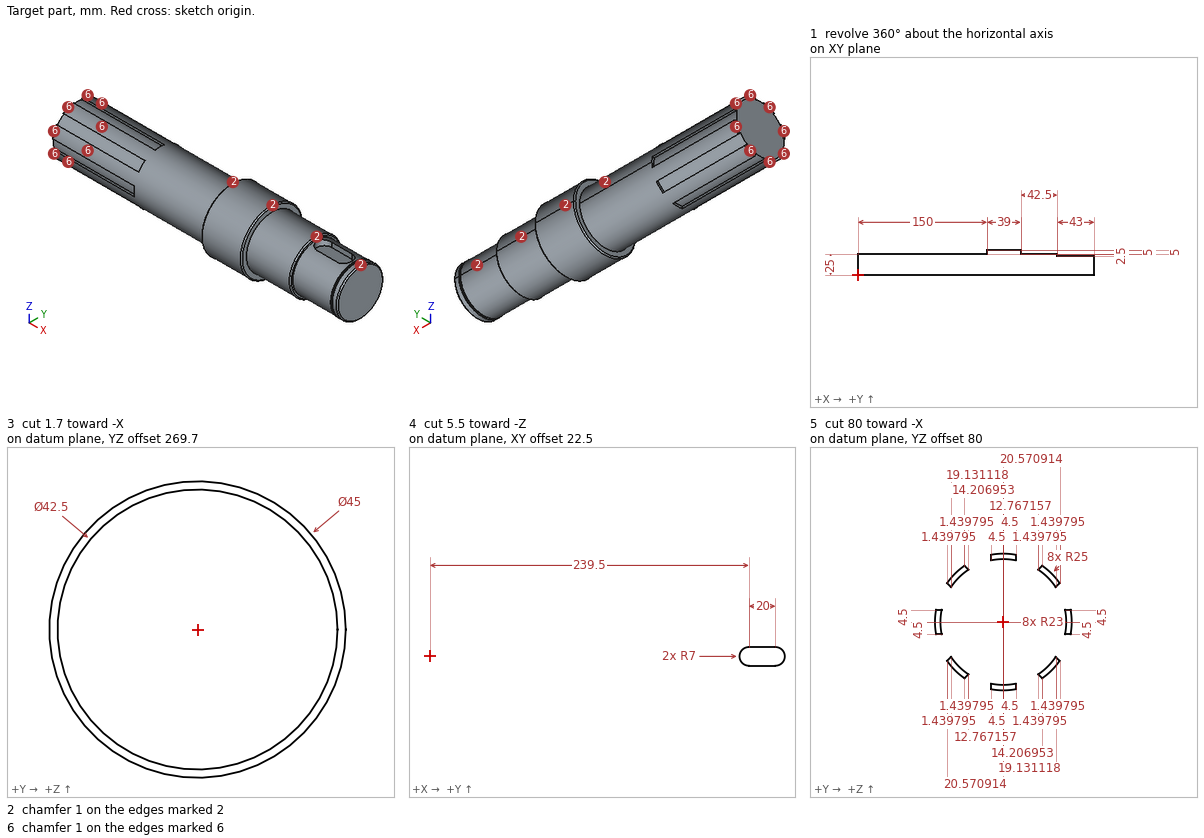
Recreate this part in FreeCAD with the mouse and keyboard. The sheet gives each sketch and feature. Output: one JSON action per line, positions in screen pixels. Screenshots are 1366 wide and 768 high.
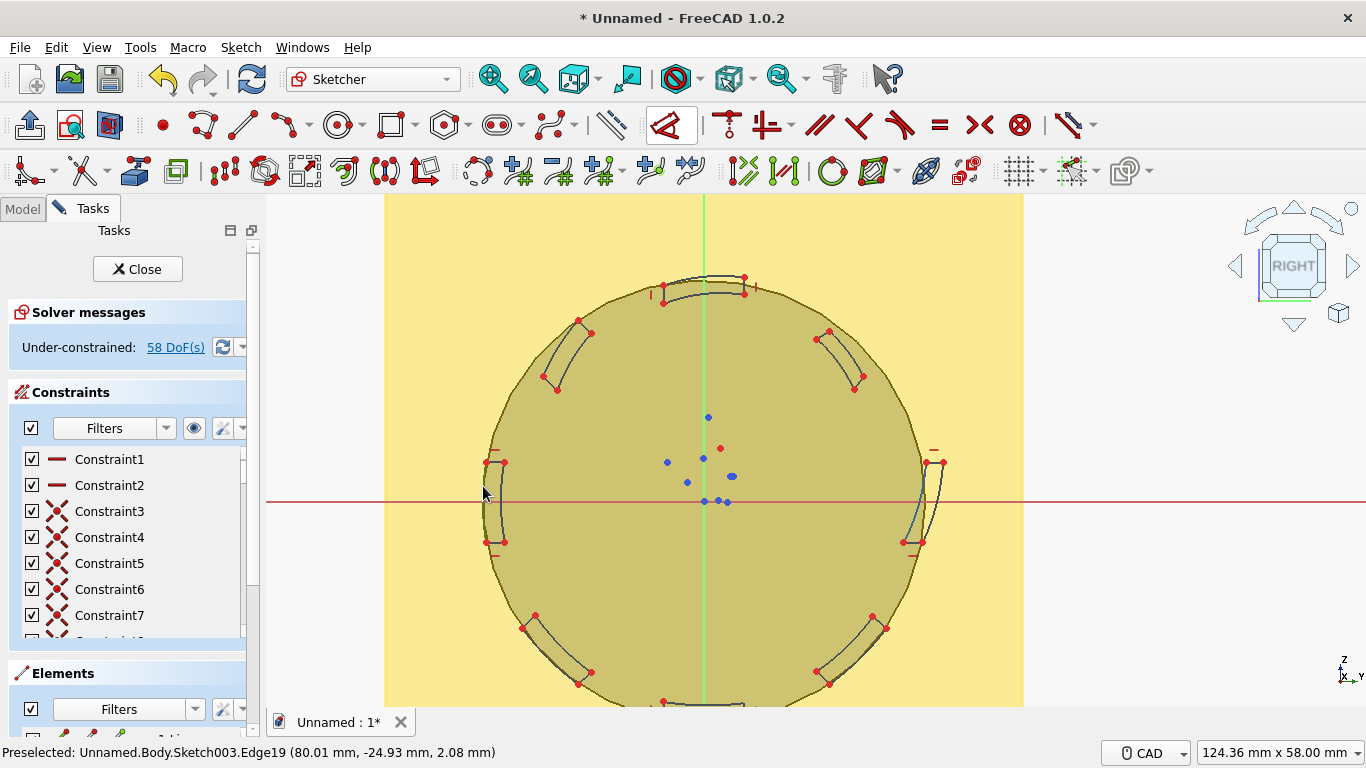
{"action": "key", "text": "c"}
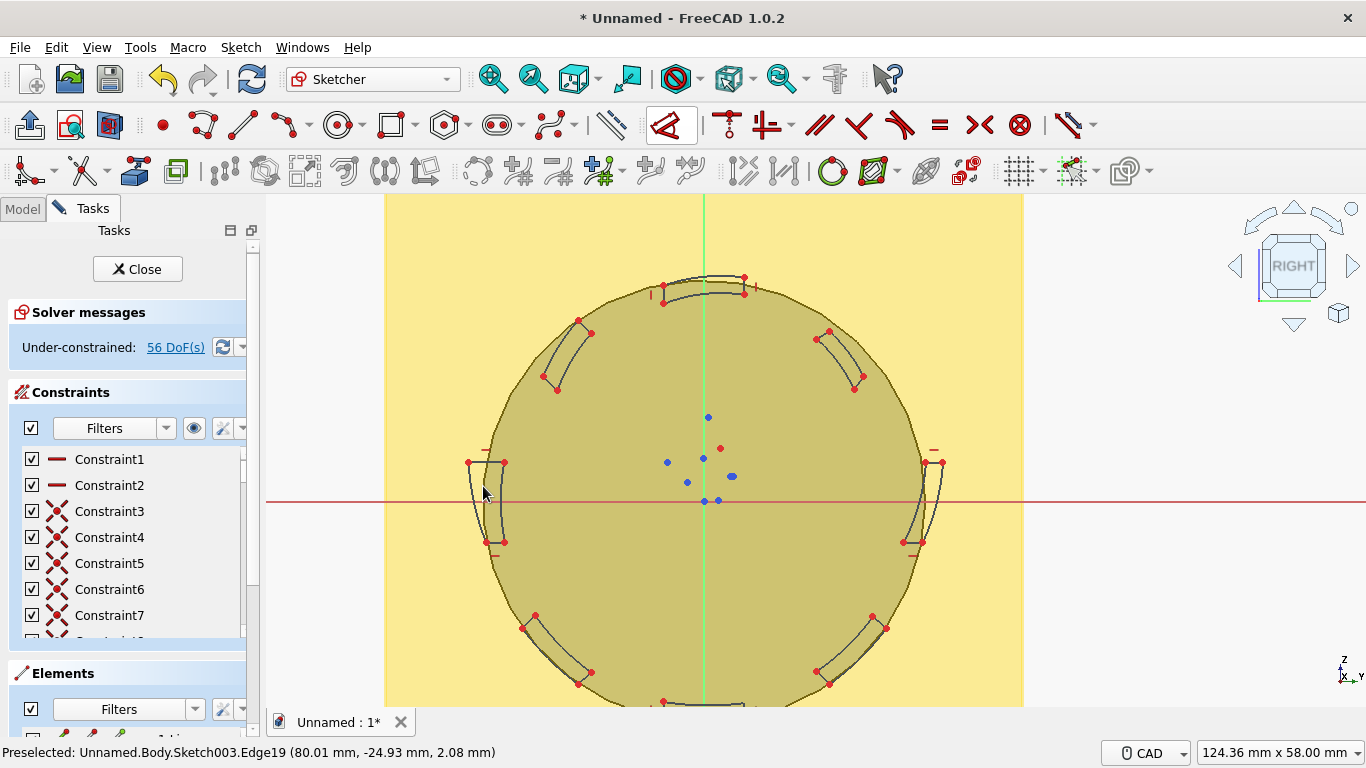
{"action": "left_click", "coordinate": [914, 520]}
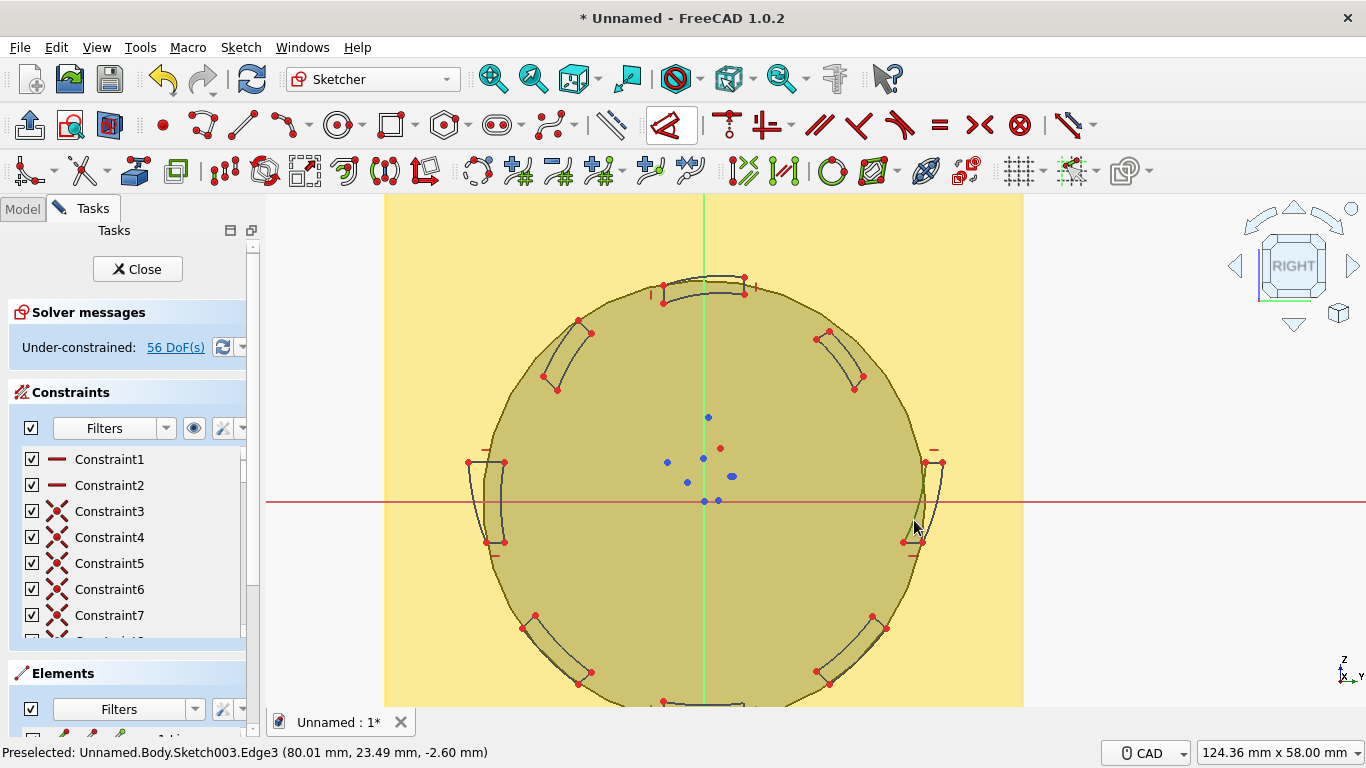
{"action": "left_click", "coordinate": [501, 486]}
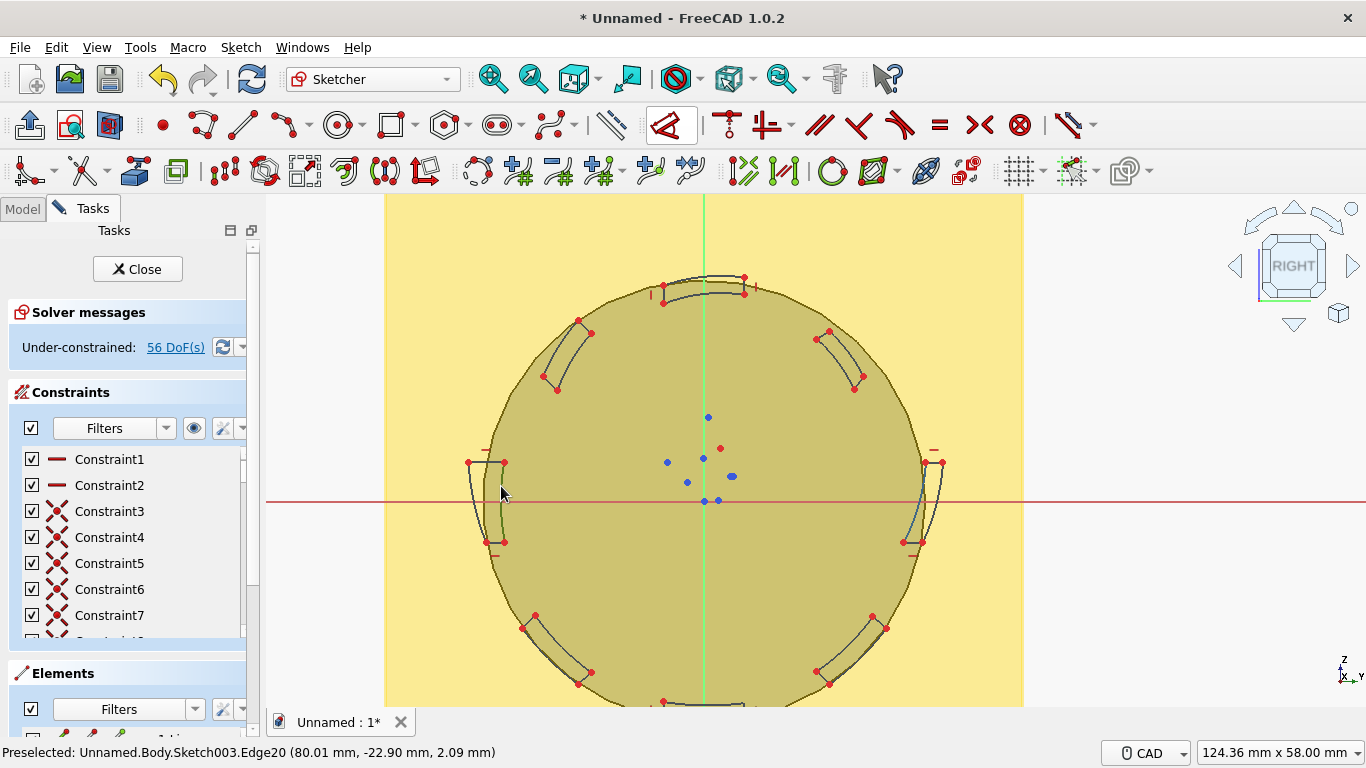
{"action": "left_click", "coordinate": [728, 126]}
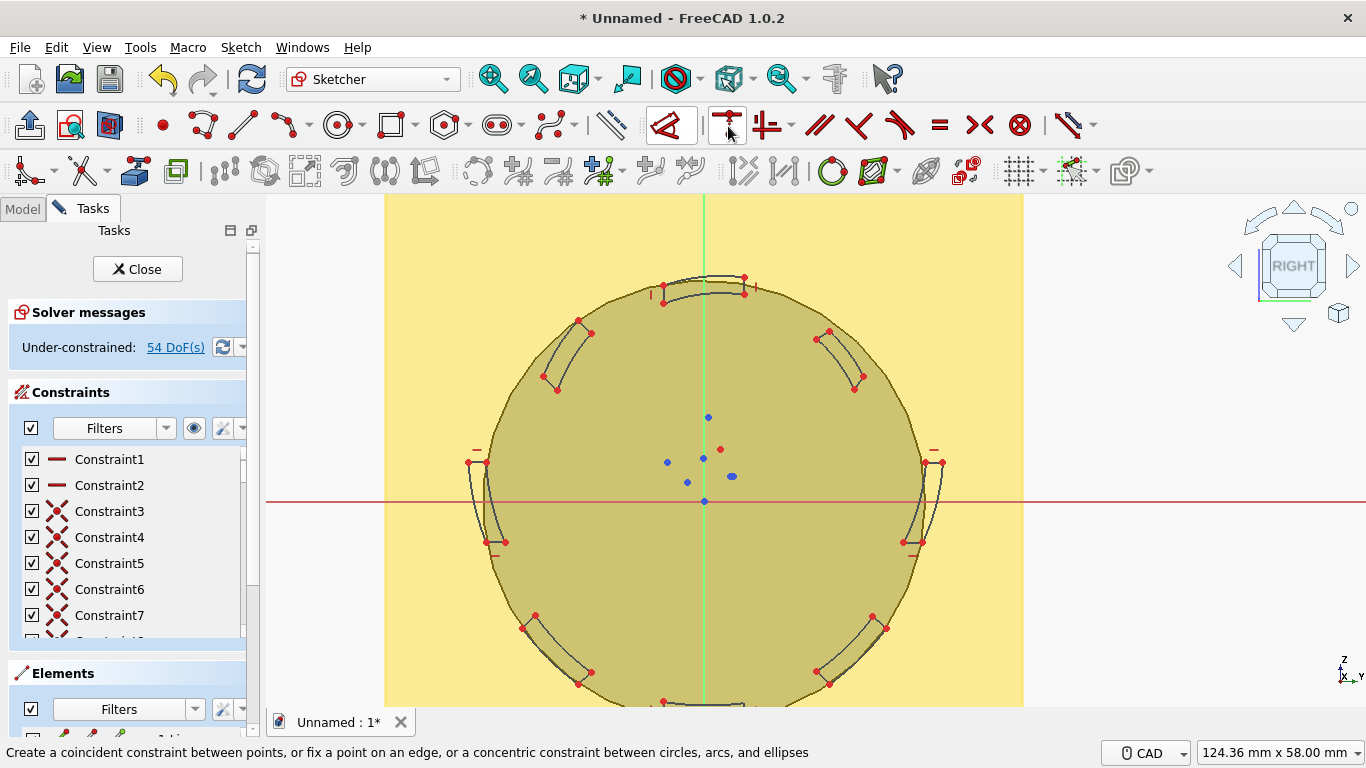
{"action": "left_click", "coordinate": [914, 520]}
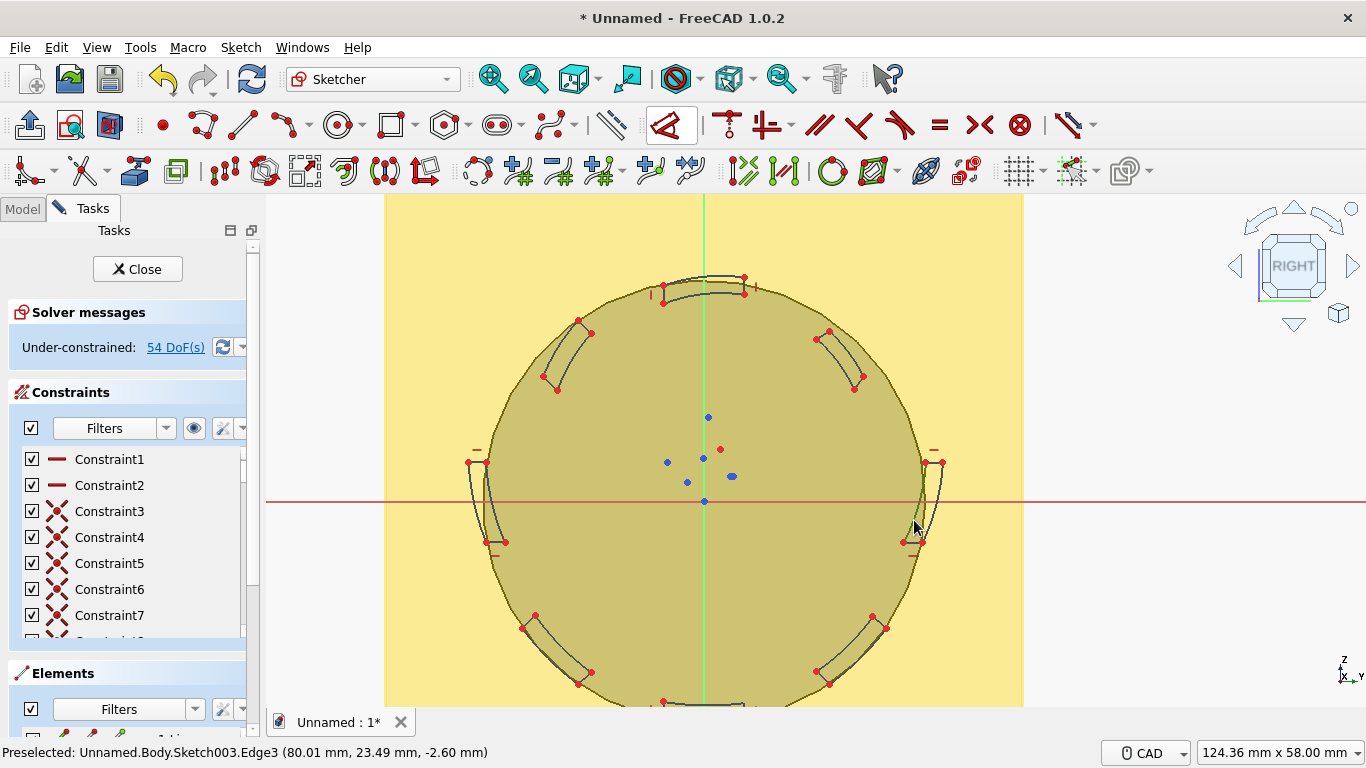
{"action": "left_click", "coordinate": [537, 647]}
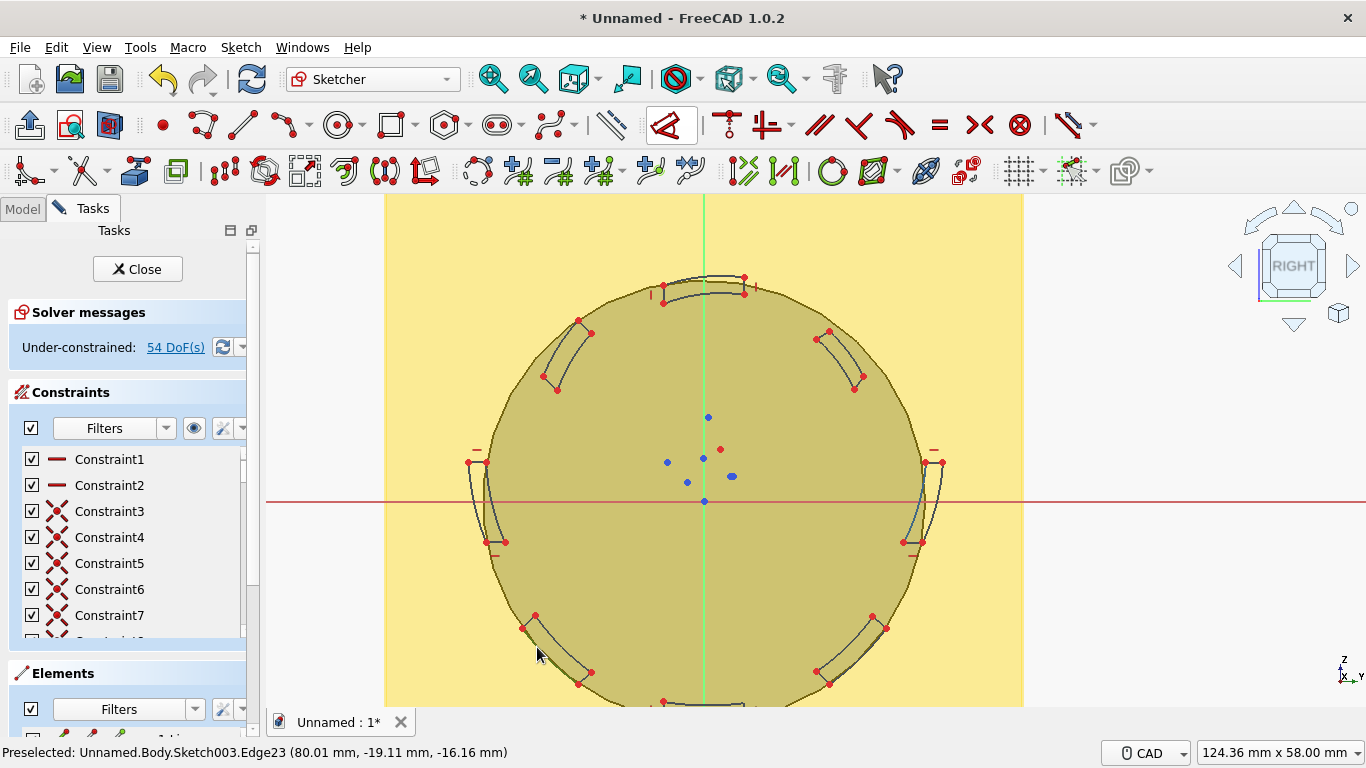
{"action": "left_click", "coordinate": [728, 126]}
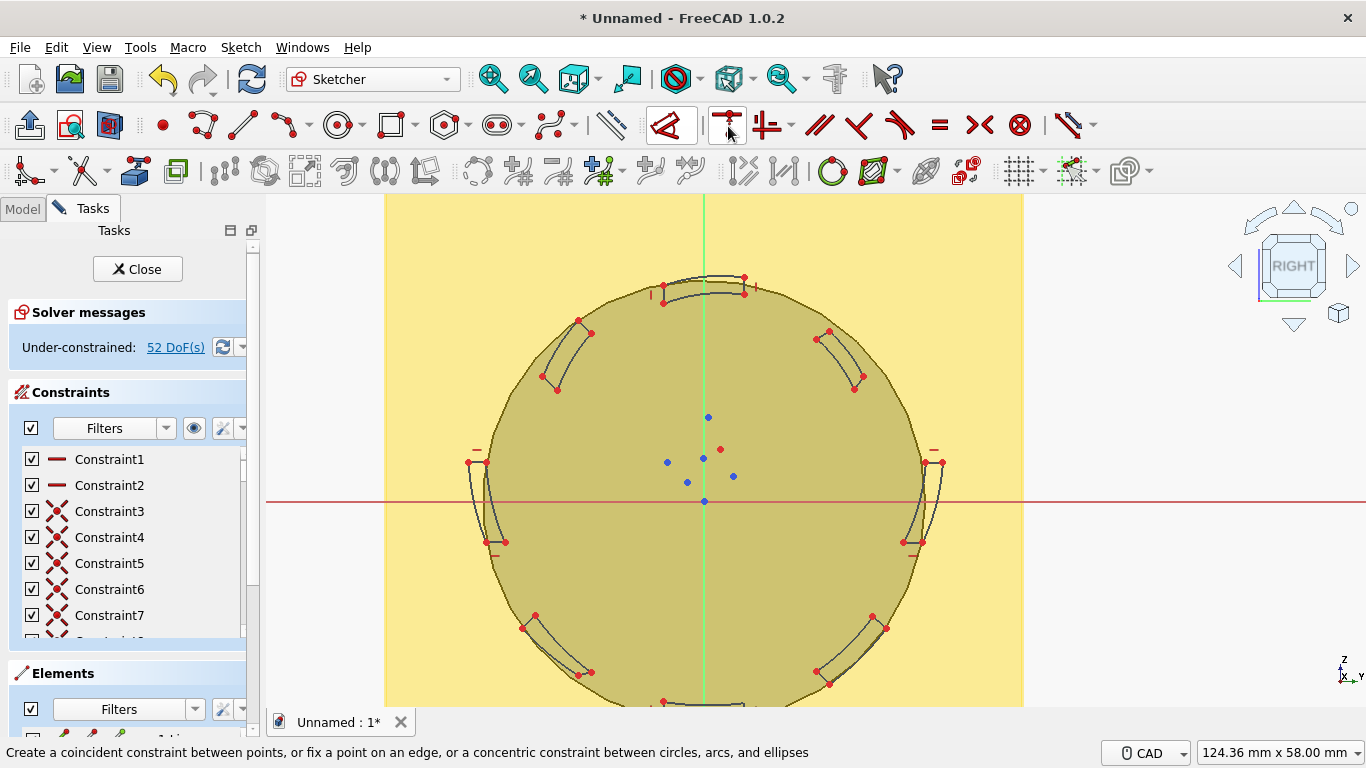
{"action": "left_click", "coordinate": [914, 520]}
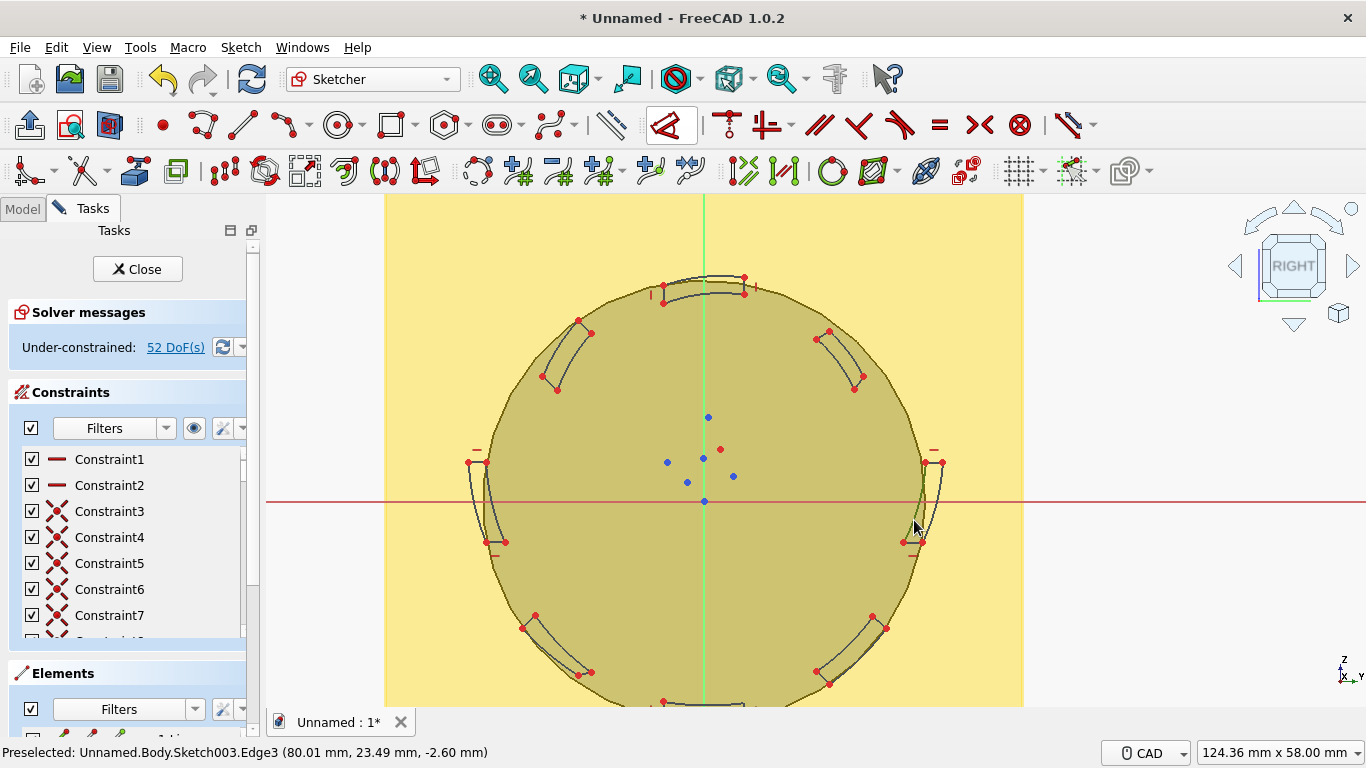
{"action": "left_click", "coordinate": [550, 634]}